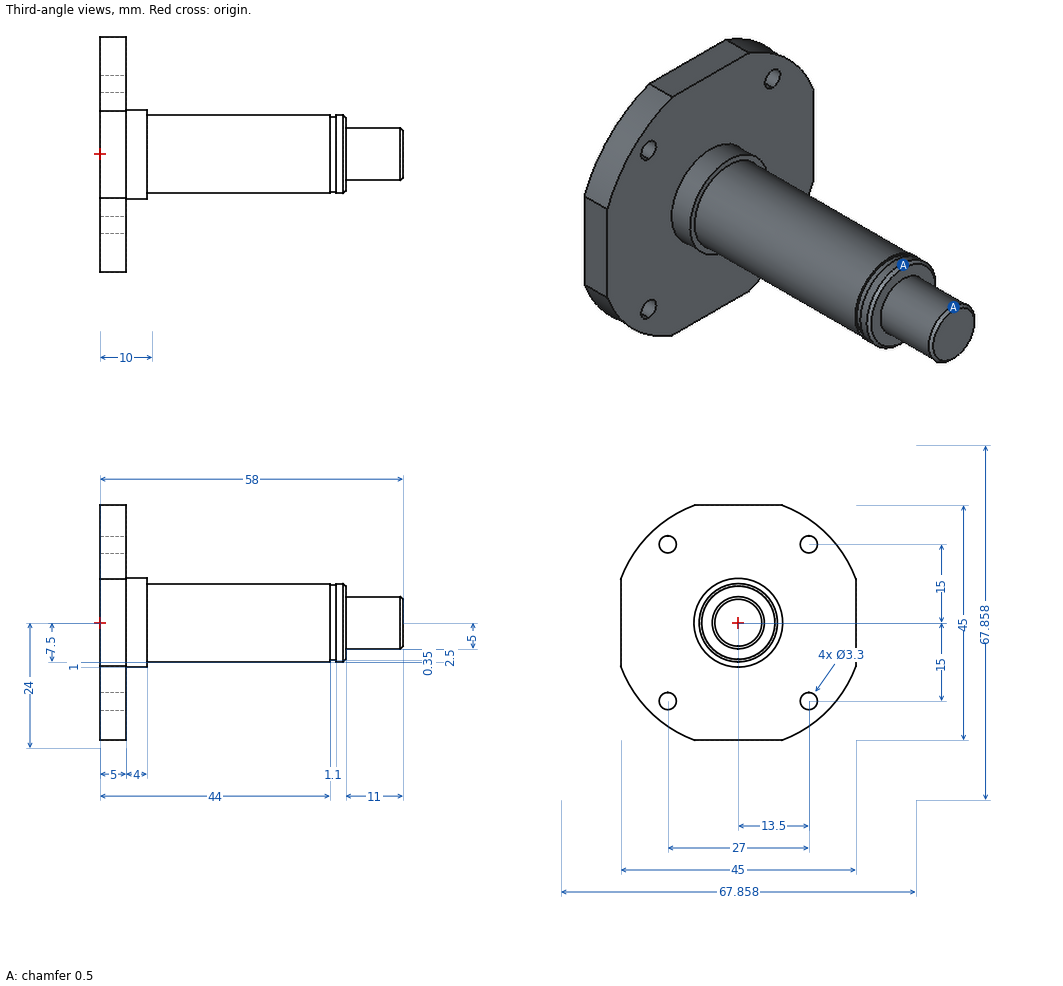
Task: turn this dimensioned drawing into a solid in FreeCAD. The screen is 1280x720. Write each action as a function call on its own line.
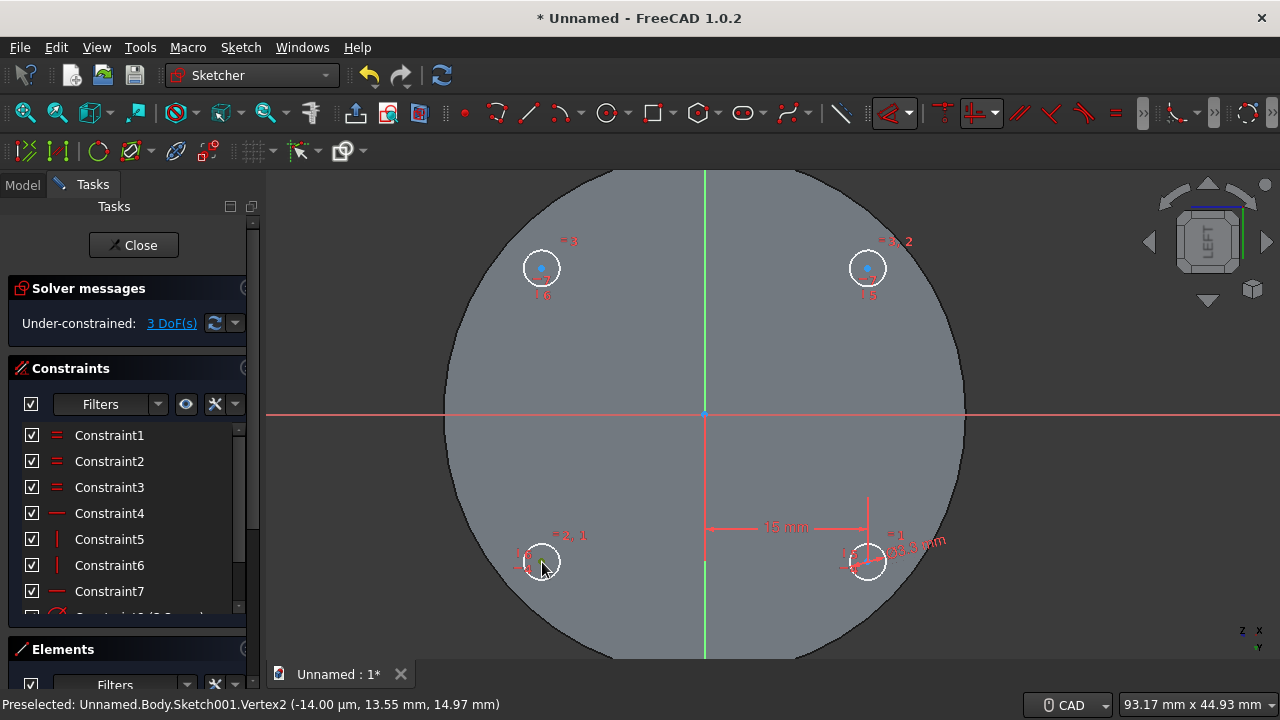
click(912, 114)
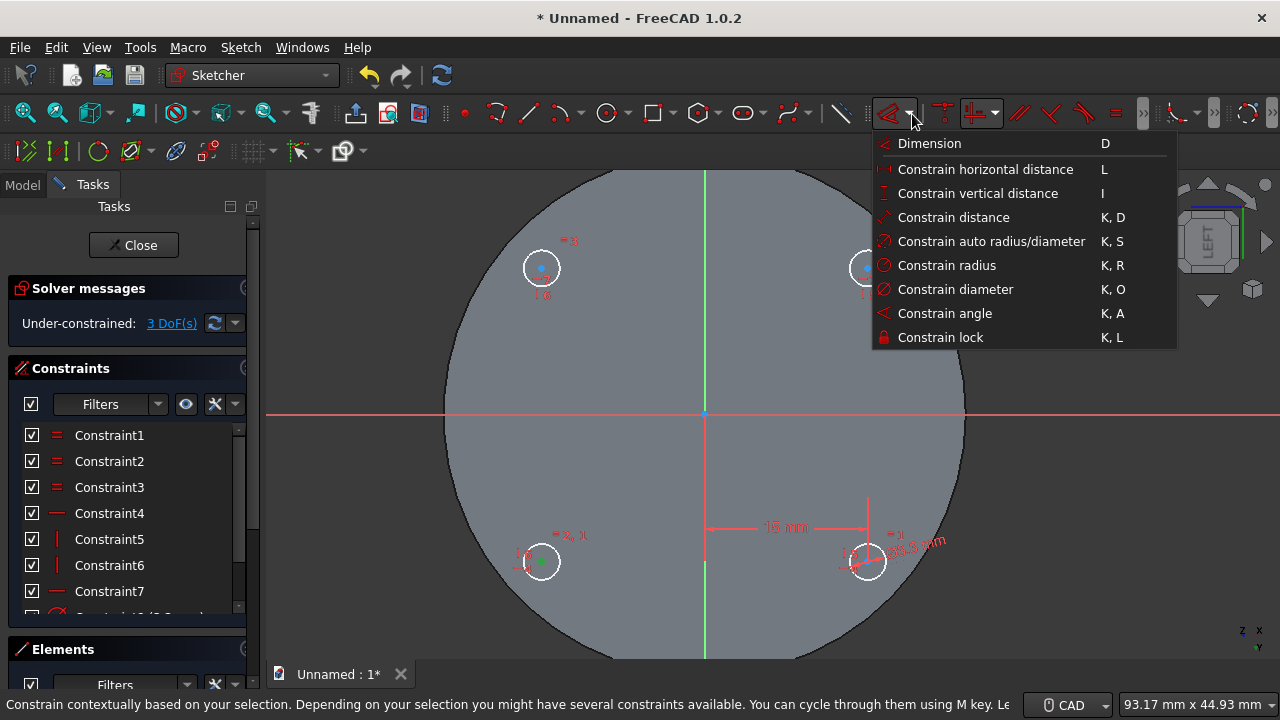
click(1025, 169)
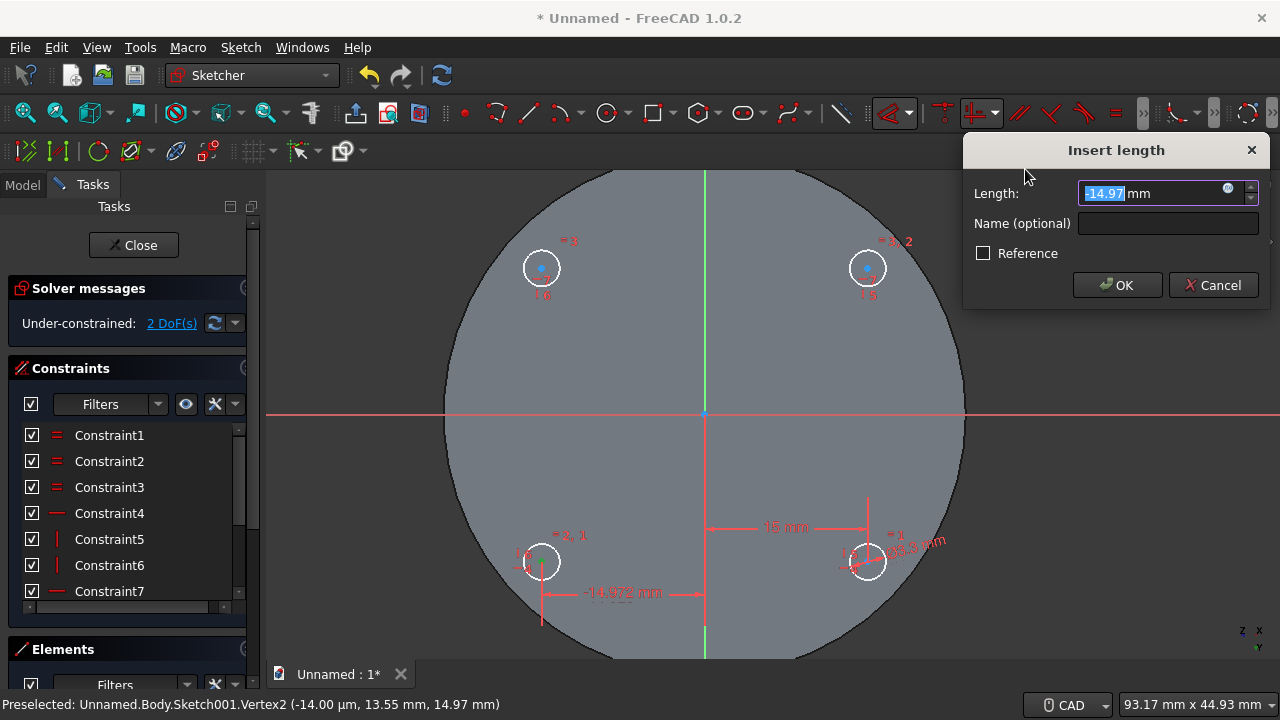
text(-15)
key(Return)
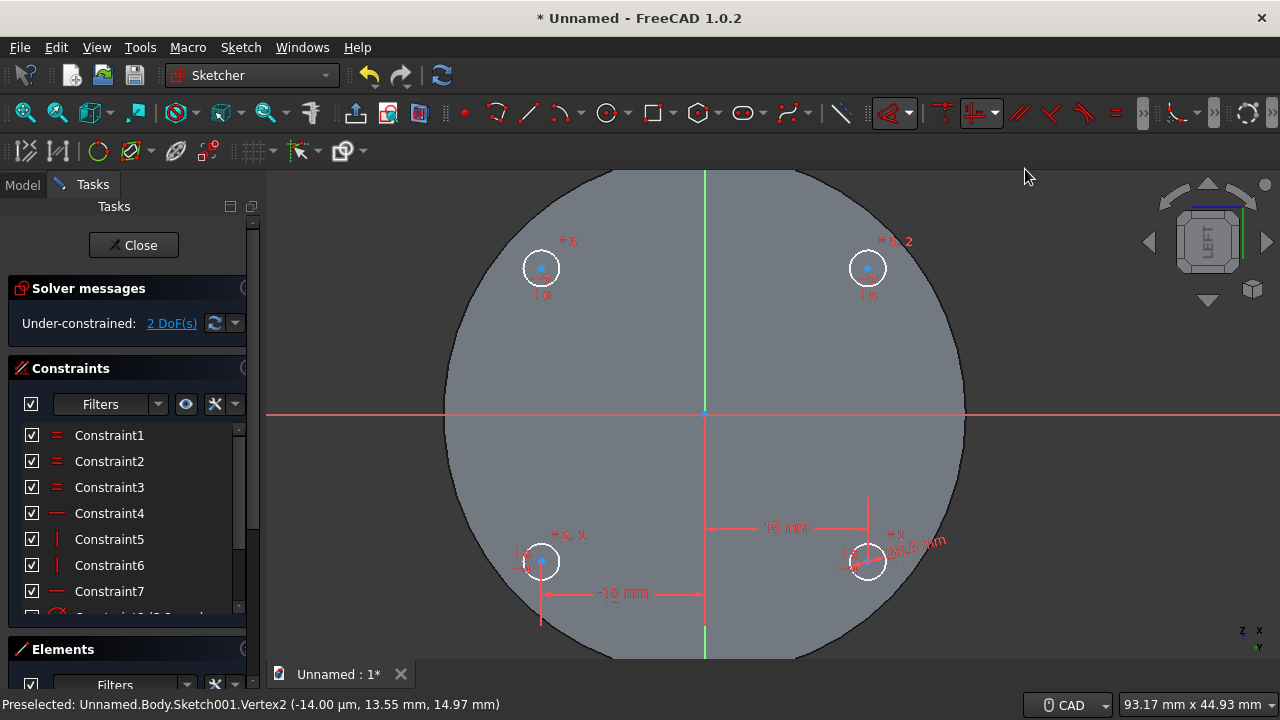
click(868, 562)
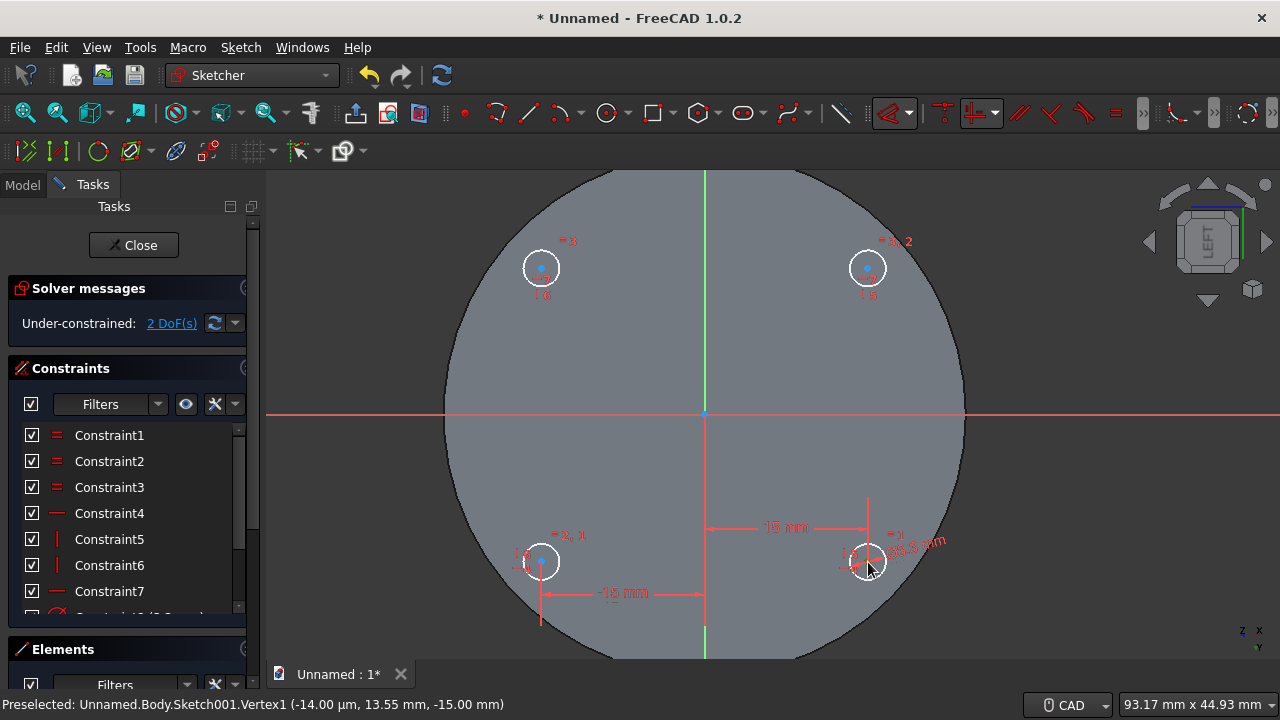
click(868, 268)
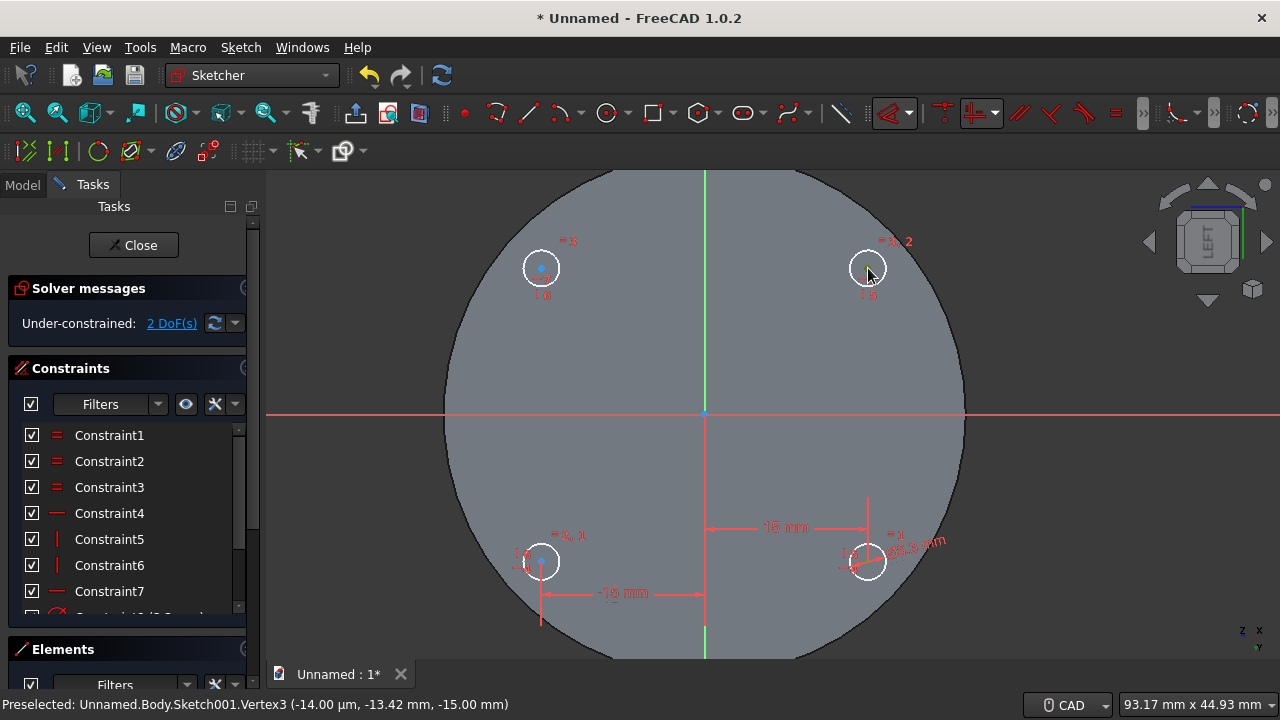
key(i)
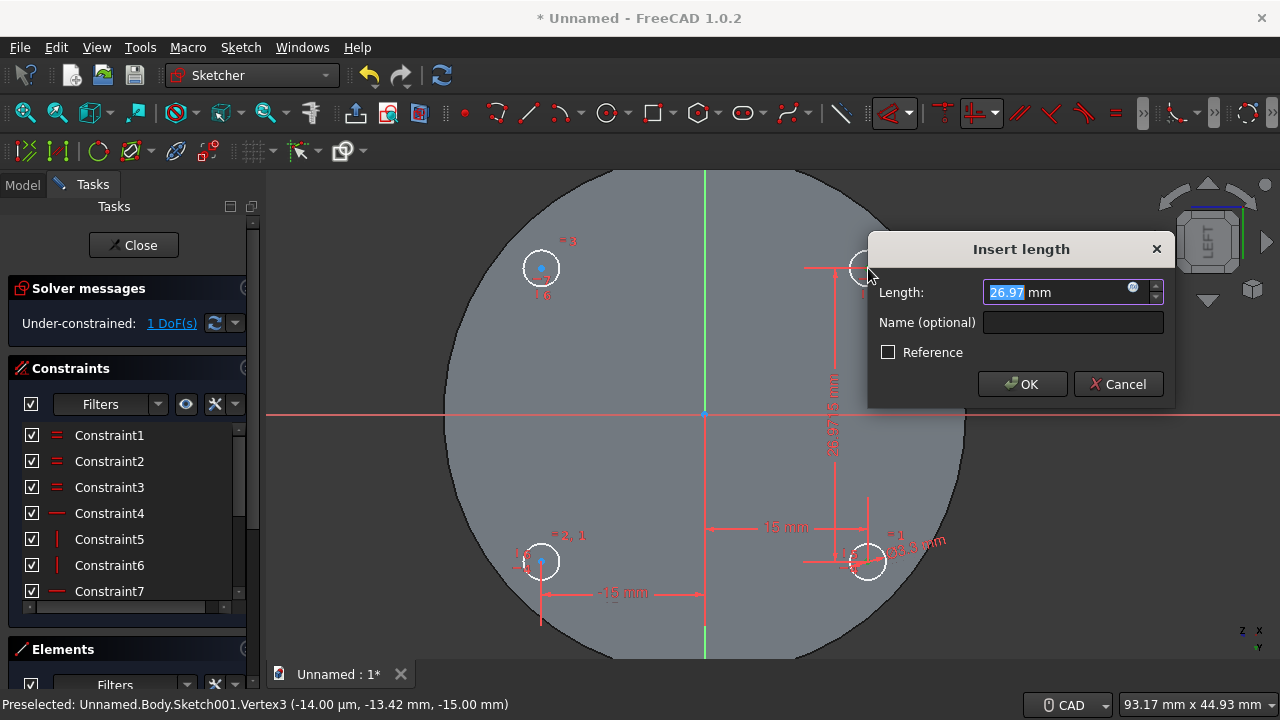
text(27)
key(Return)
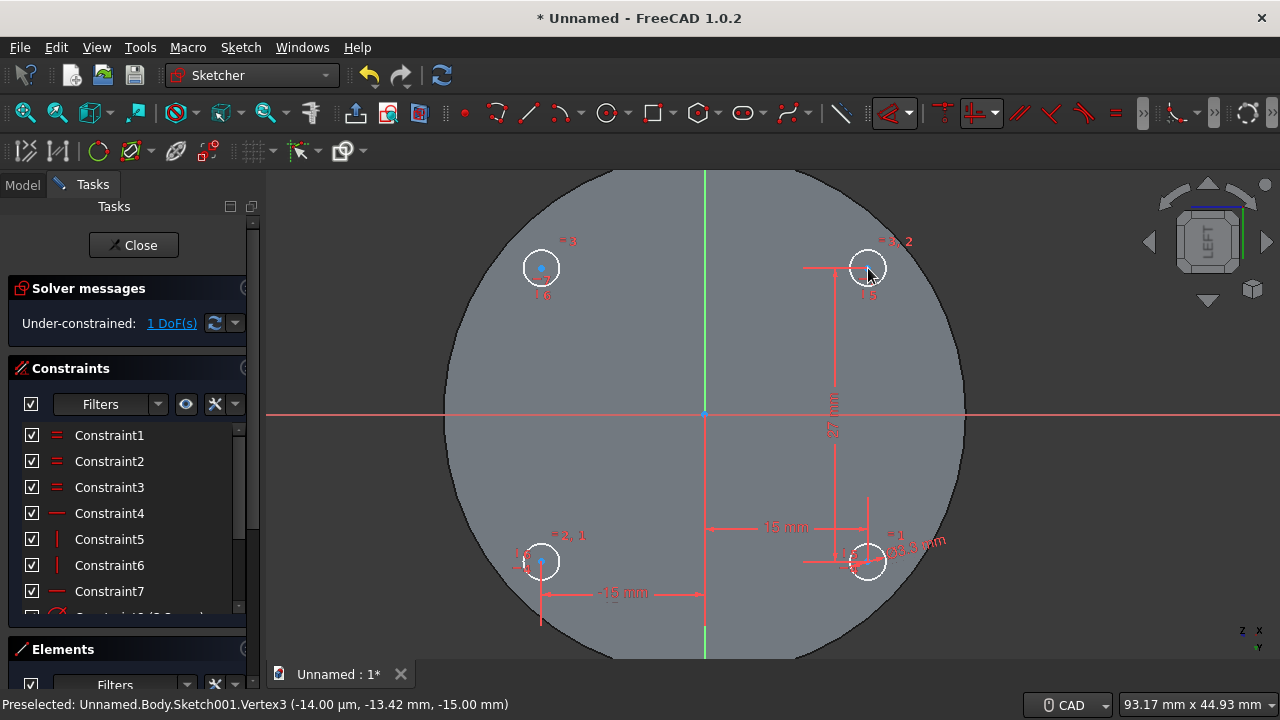
click(868, 562)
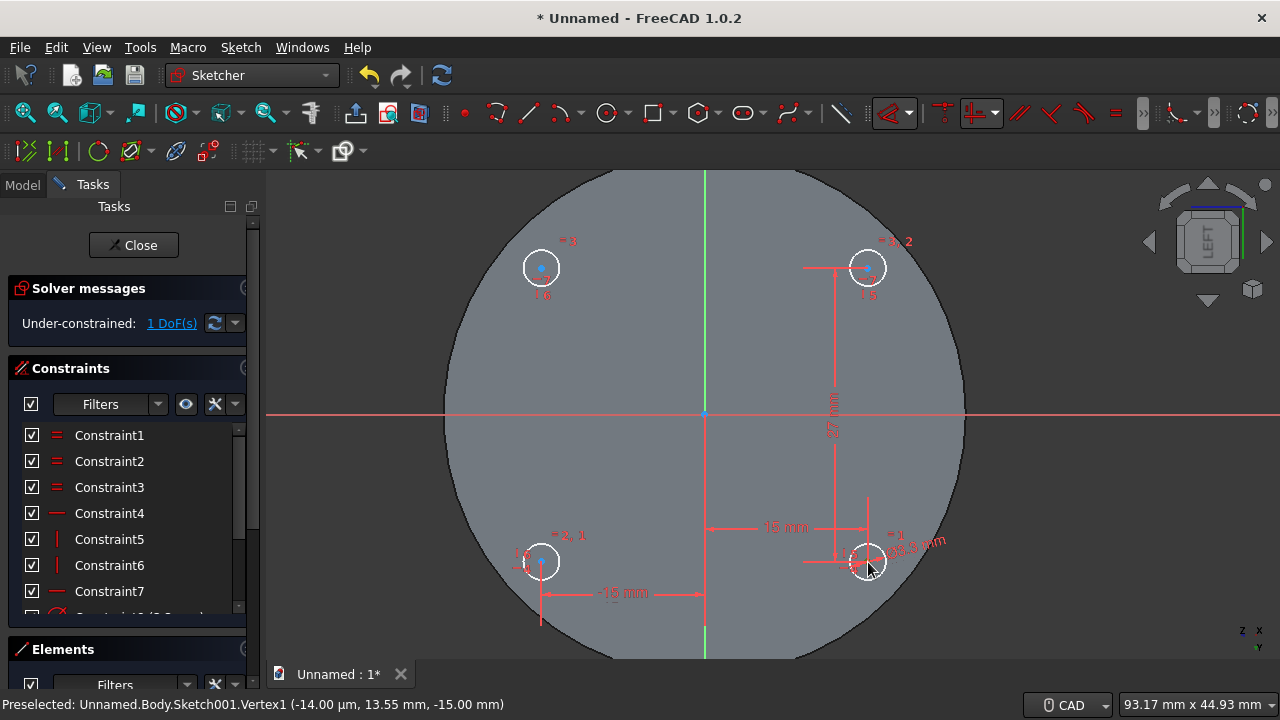
key(i)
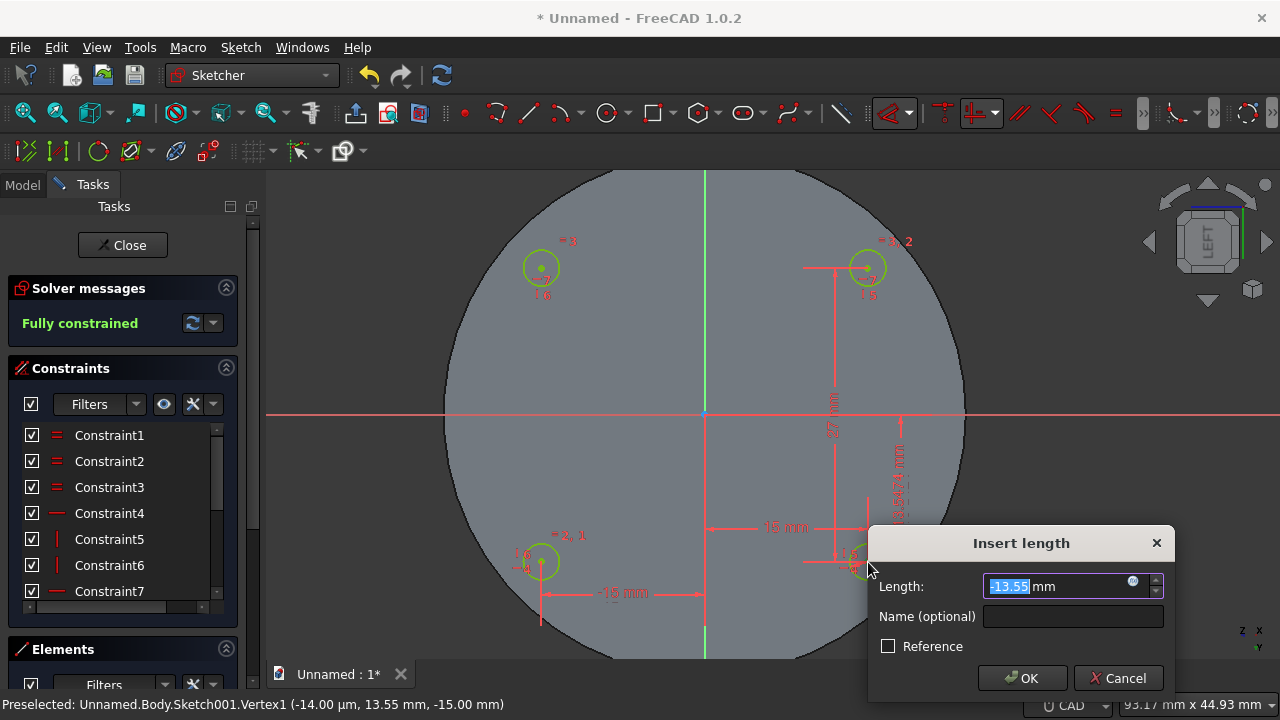
text(-13.5)
key(Return)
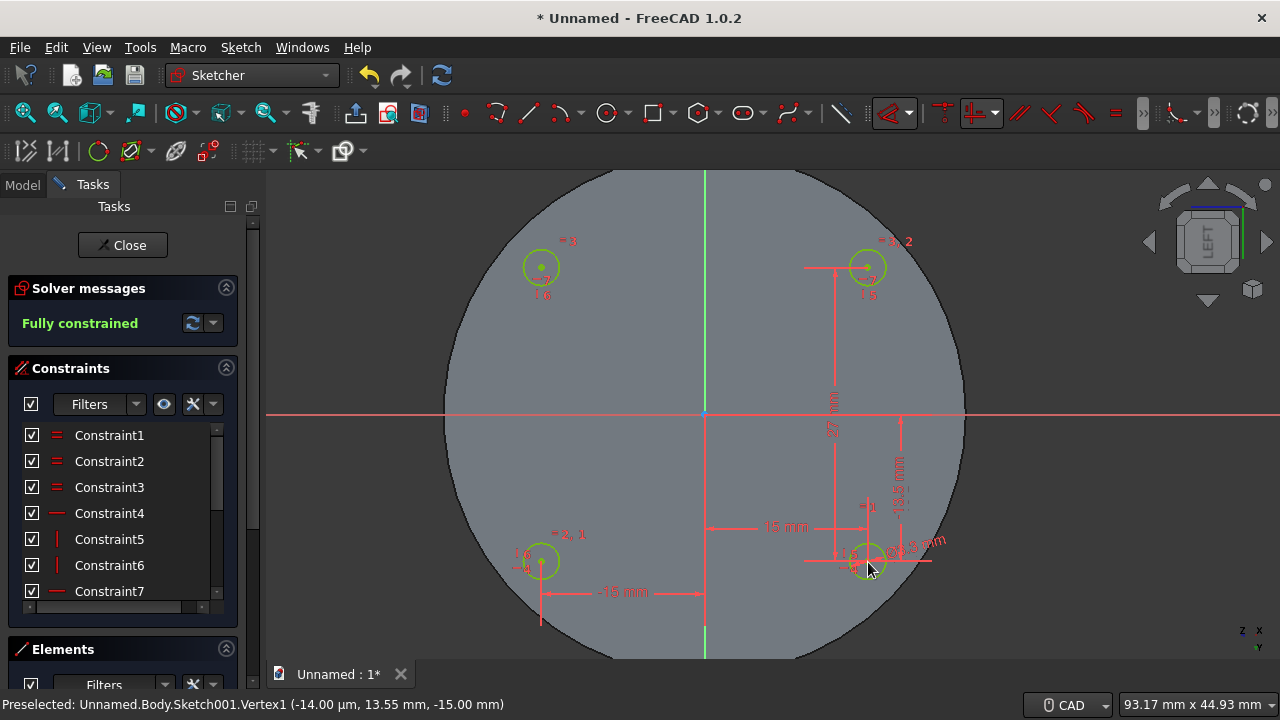
click(123, 245)